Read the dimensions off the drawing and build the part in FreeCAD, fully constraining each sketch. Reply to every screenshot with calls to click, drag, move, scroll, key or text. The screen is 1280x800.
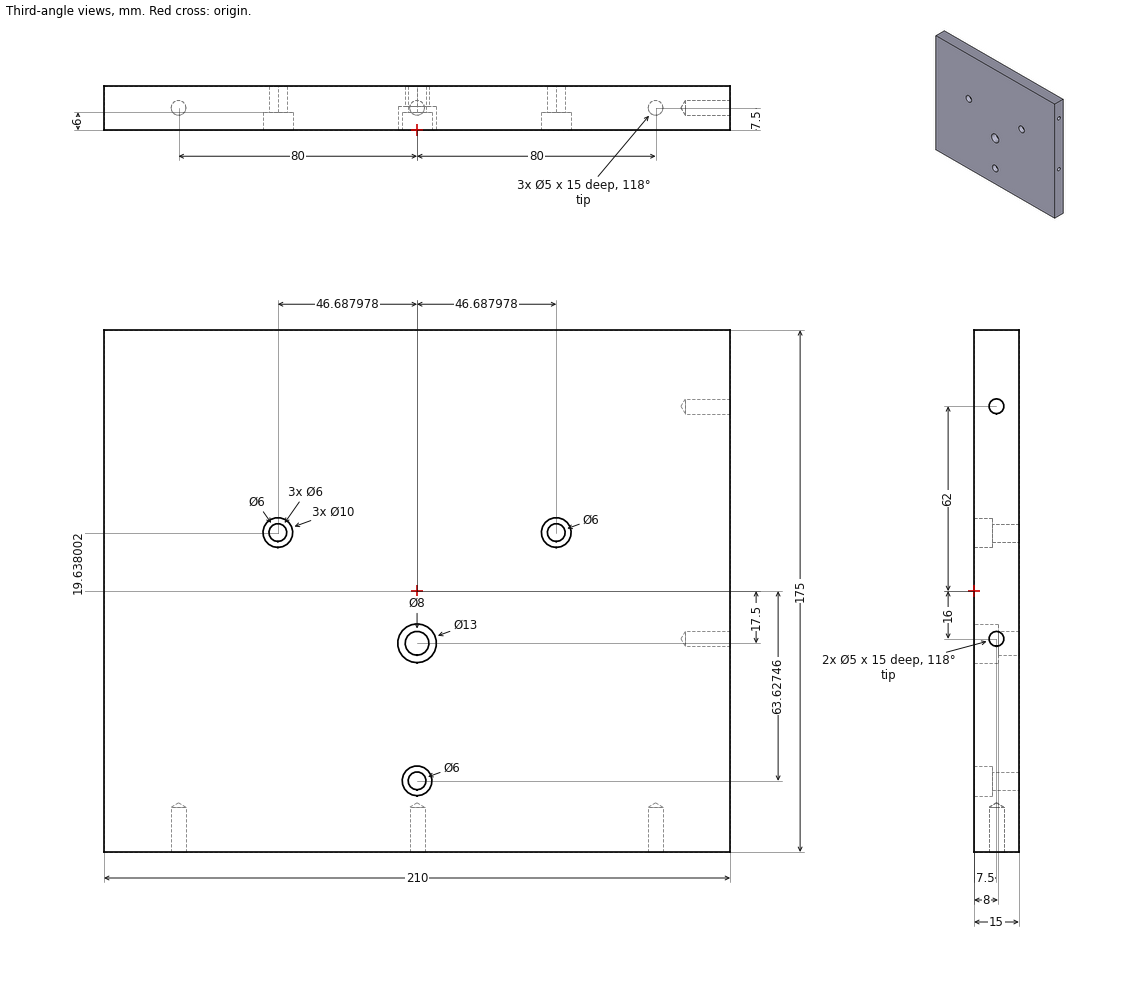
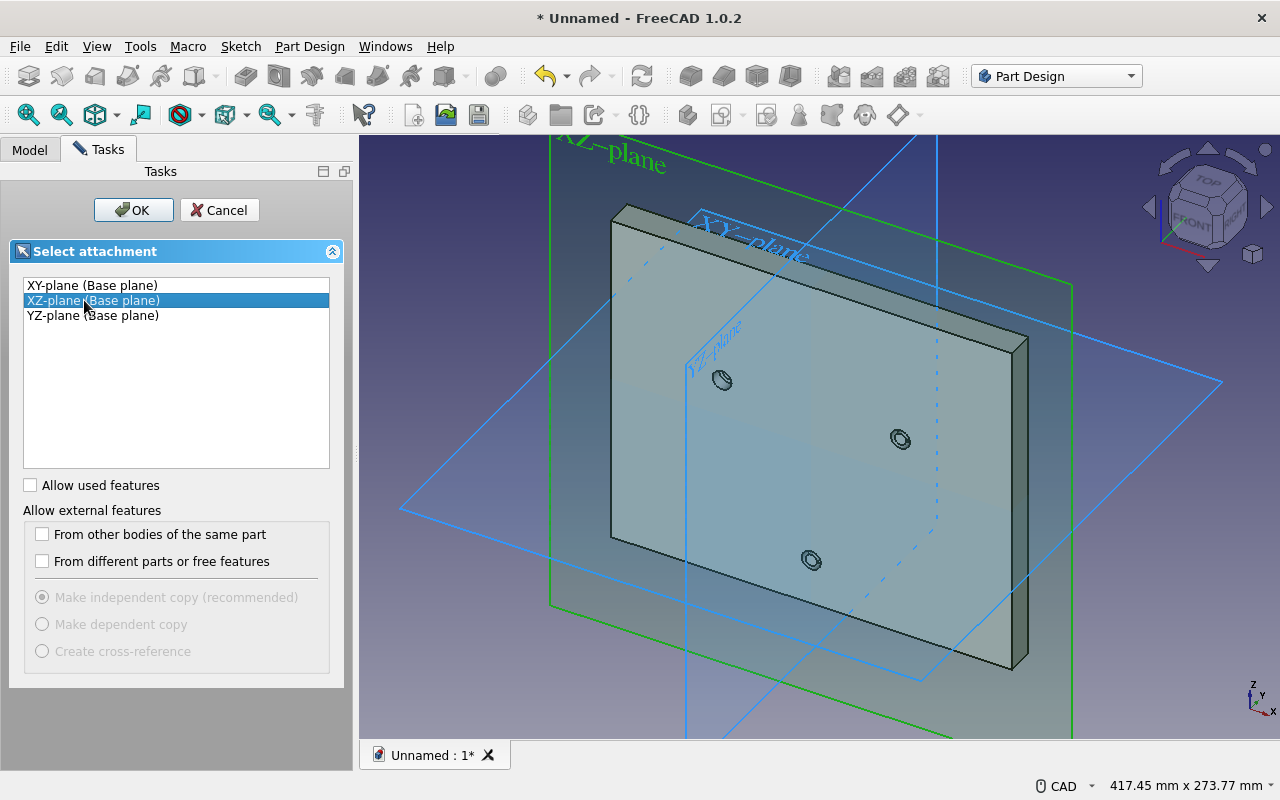
click(134, 210)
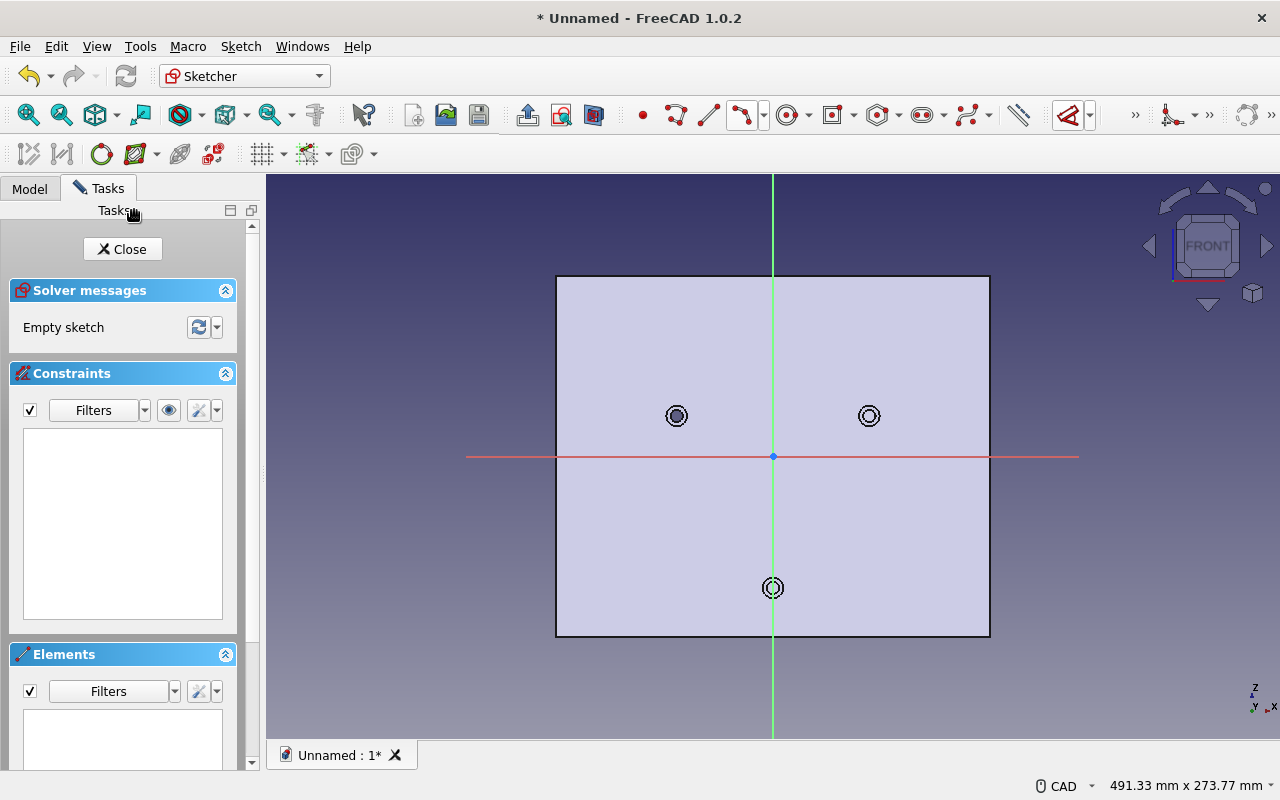
scroll(878, 414, up, 15)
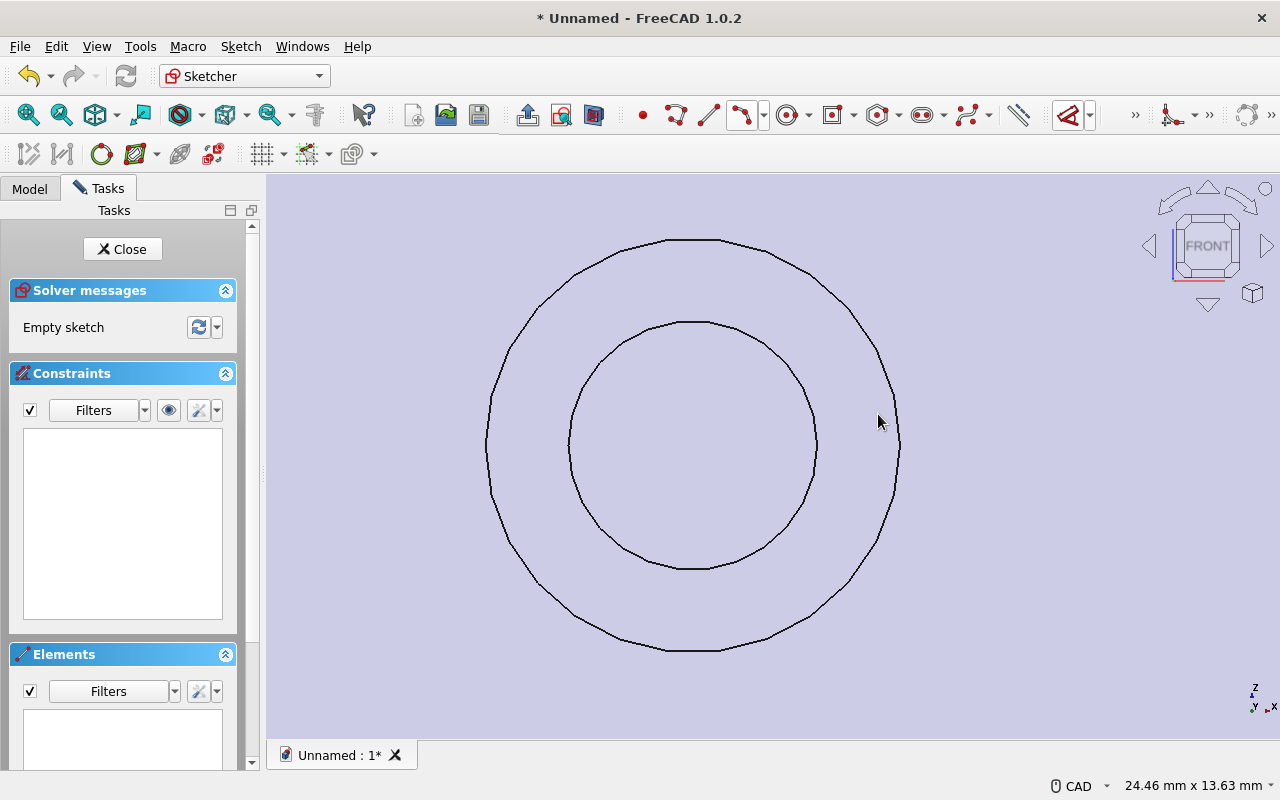
scroll(669, 423, up, 2)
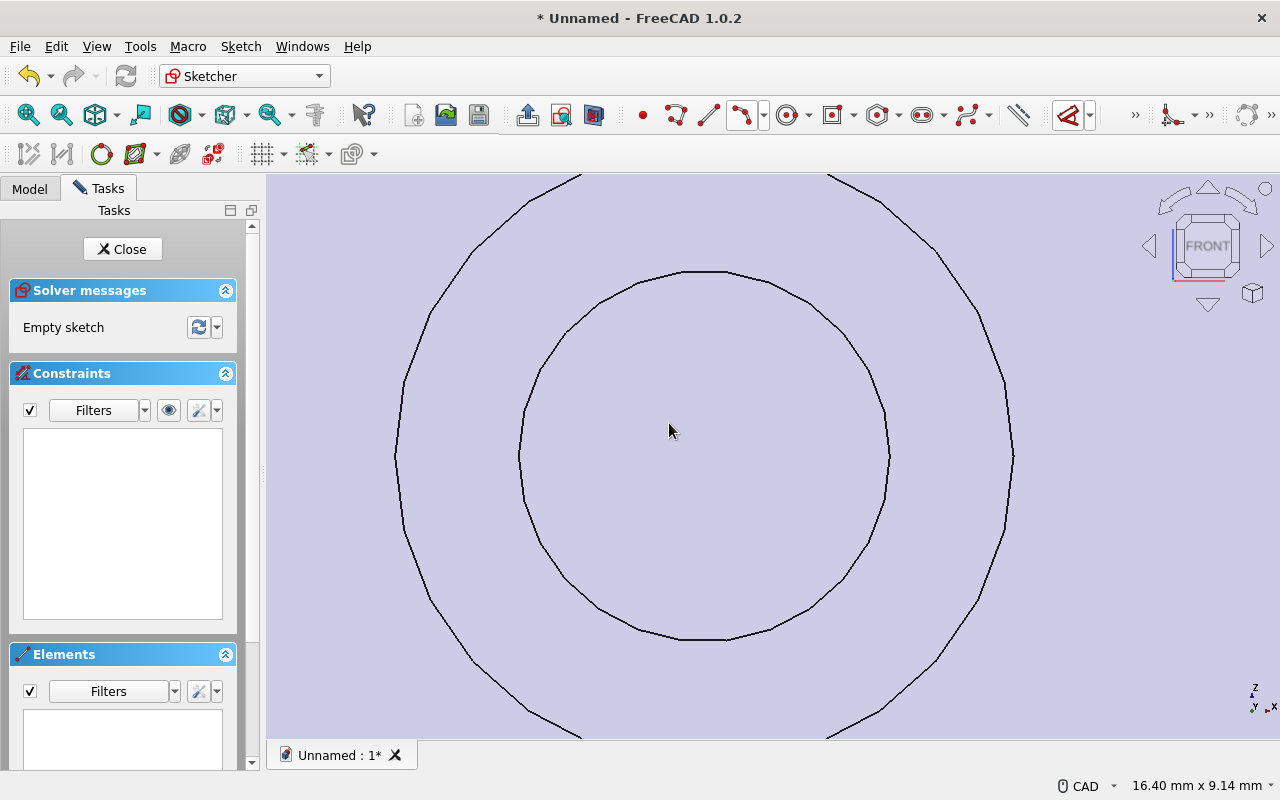
click(786, 116)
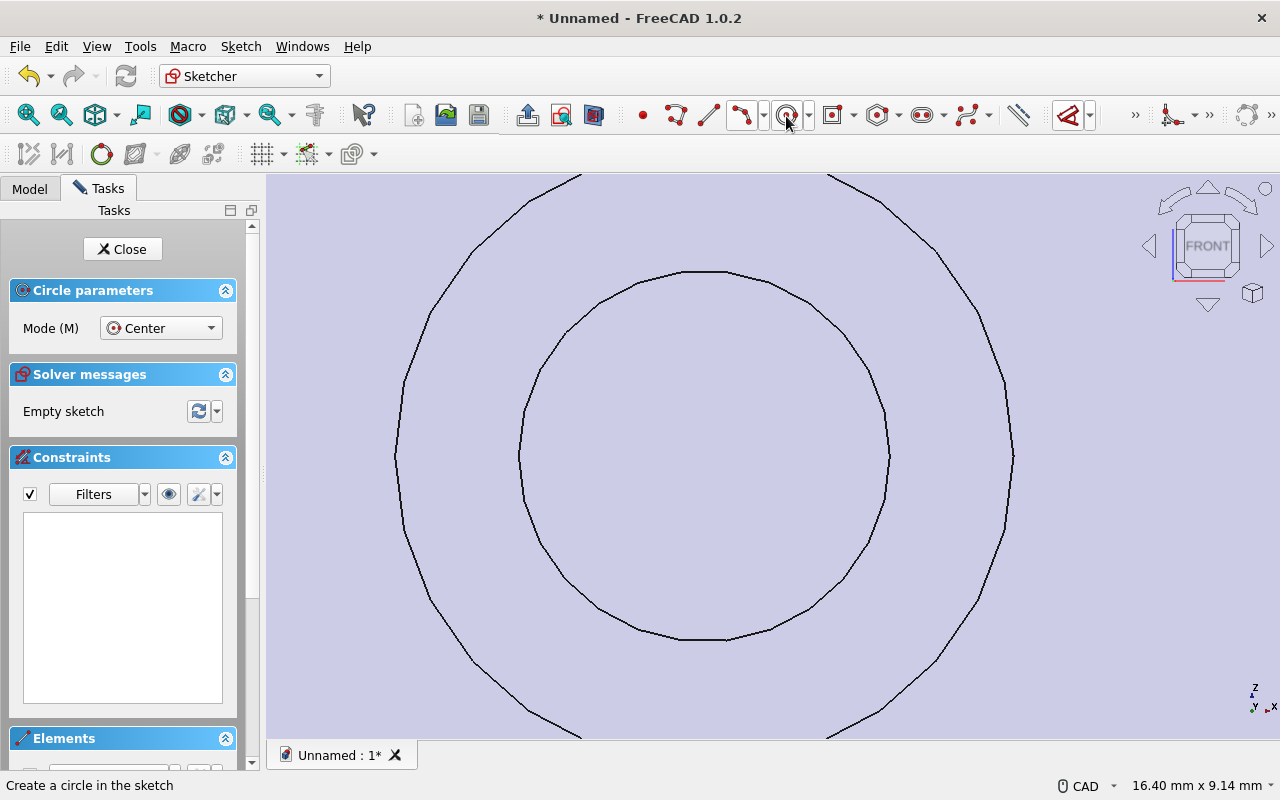
click(704, 456)
click(835, 325)
key(Escape)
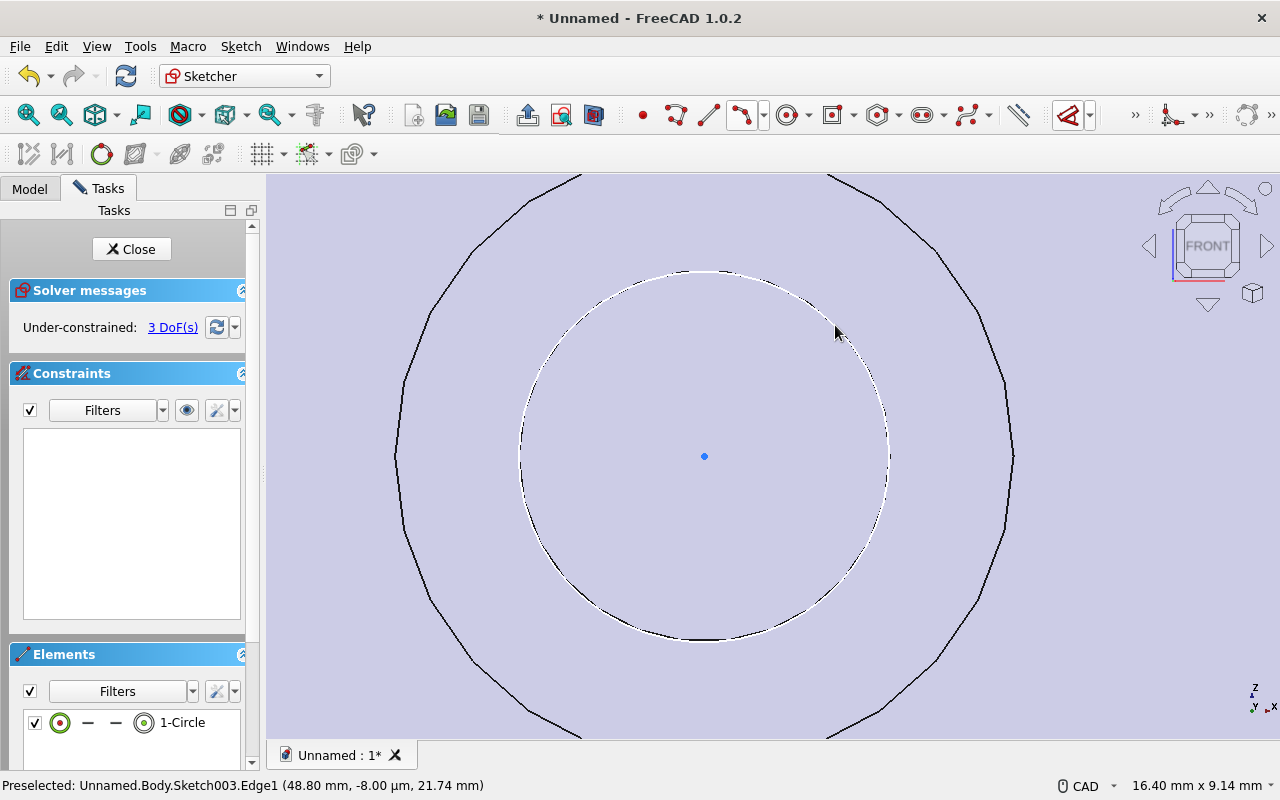
click(835, 326)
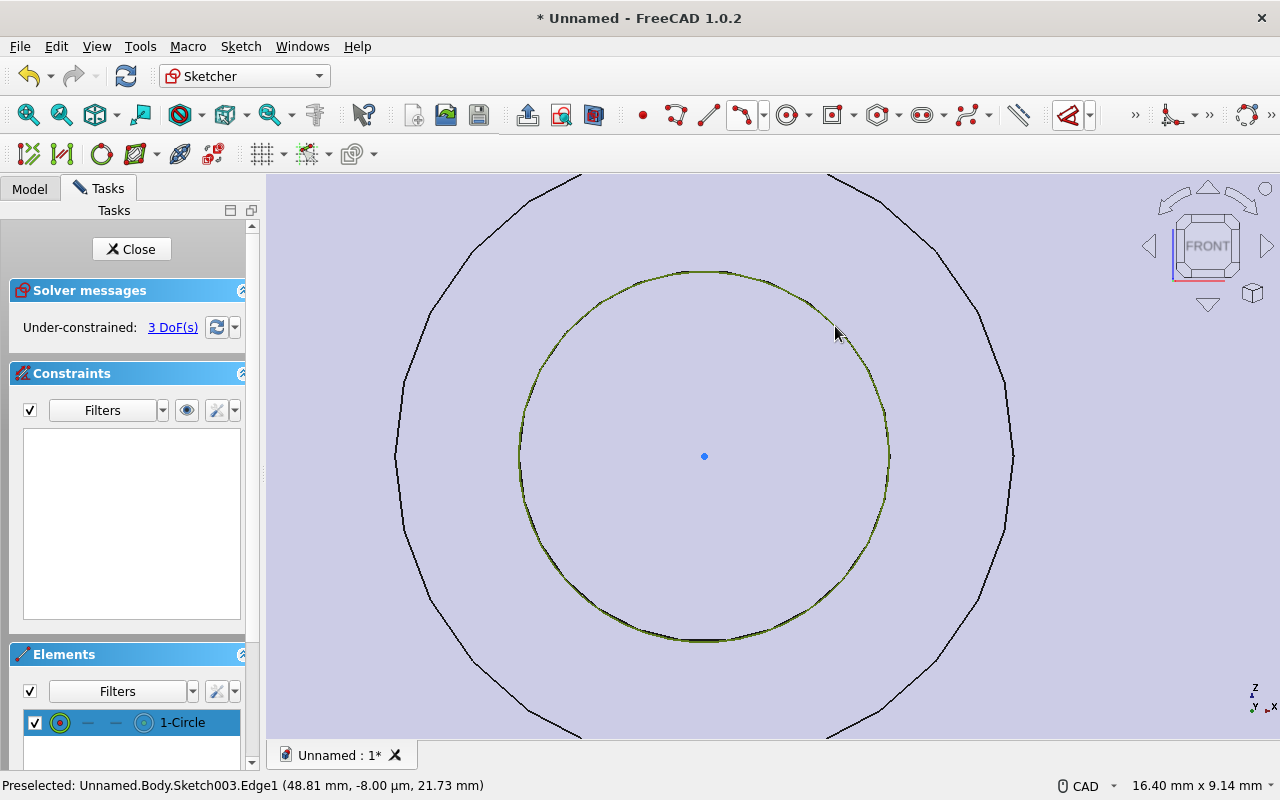
key(k)
key(o)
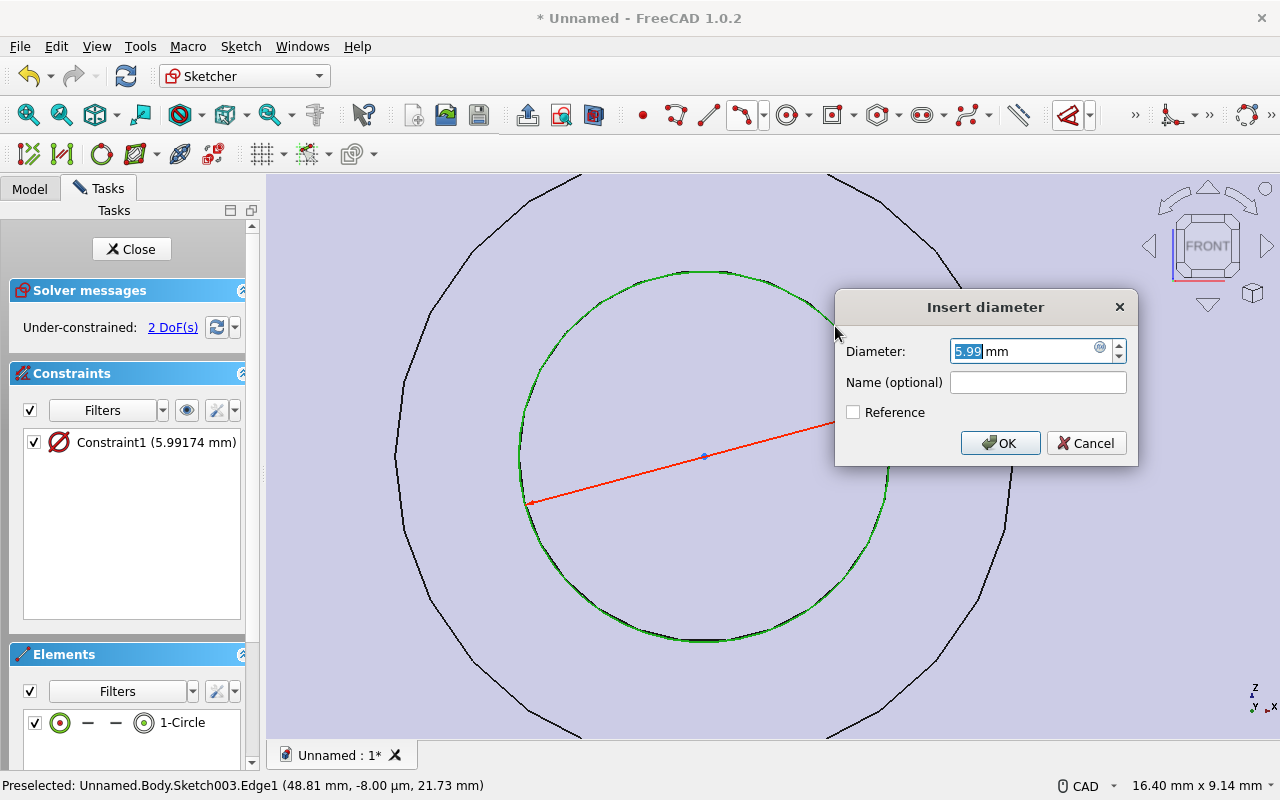
text(6)
key(Return)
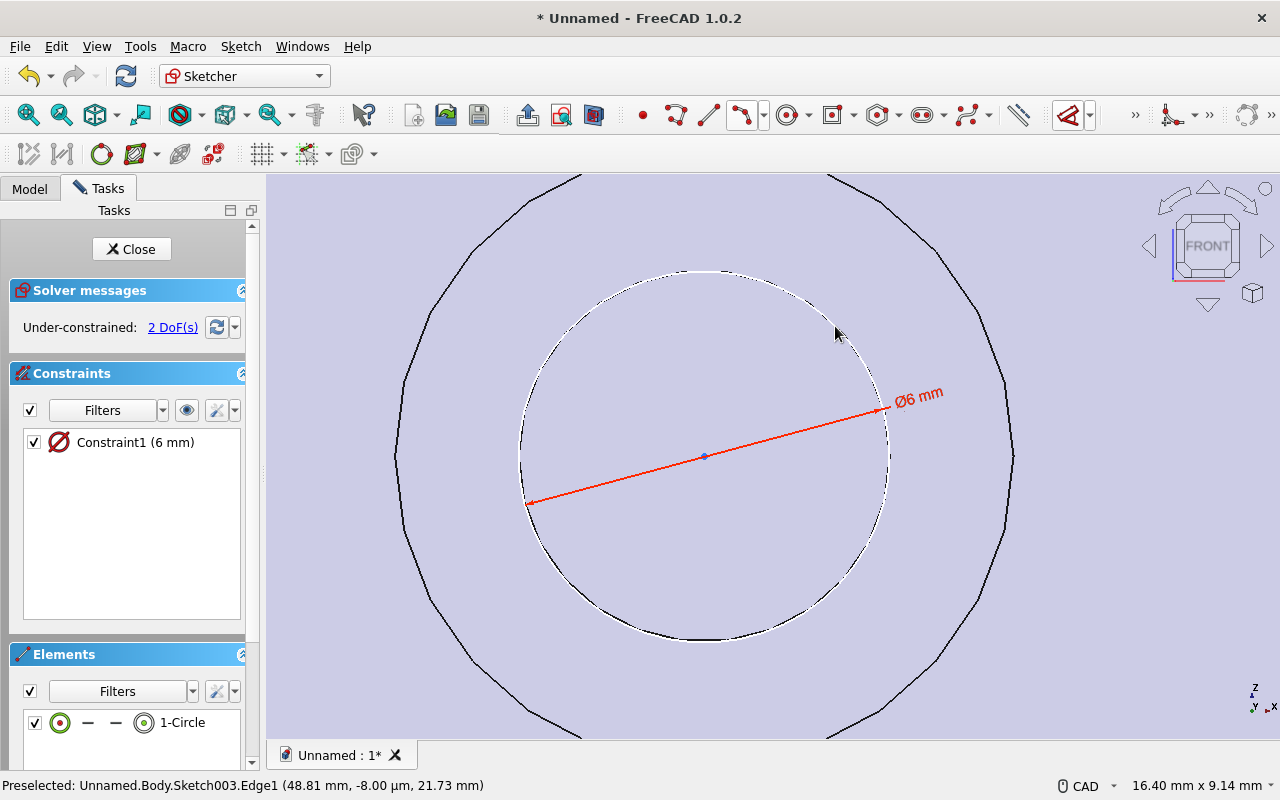
click(704, 457)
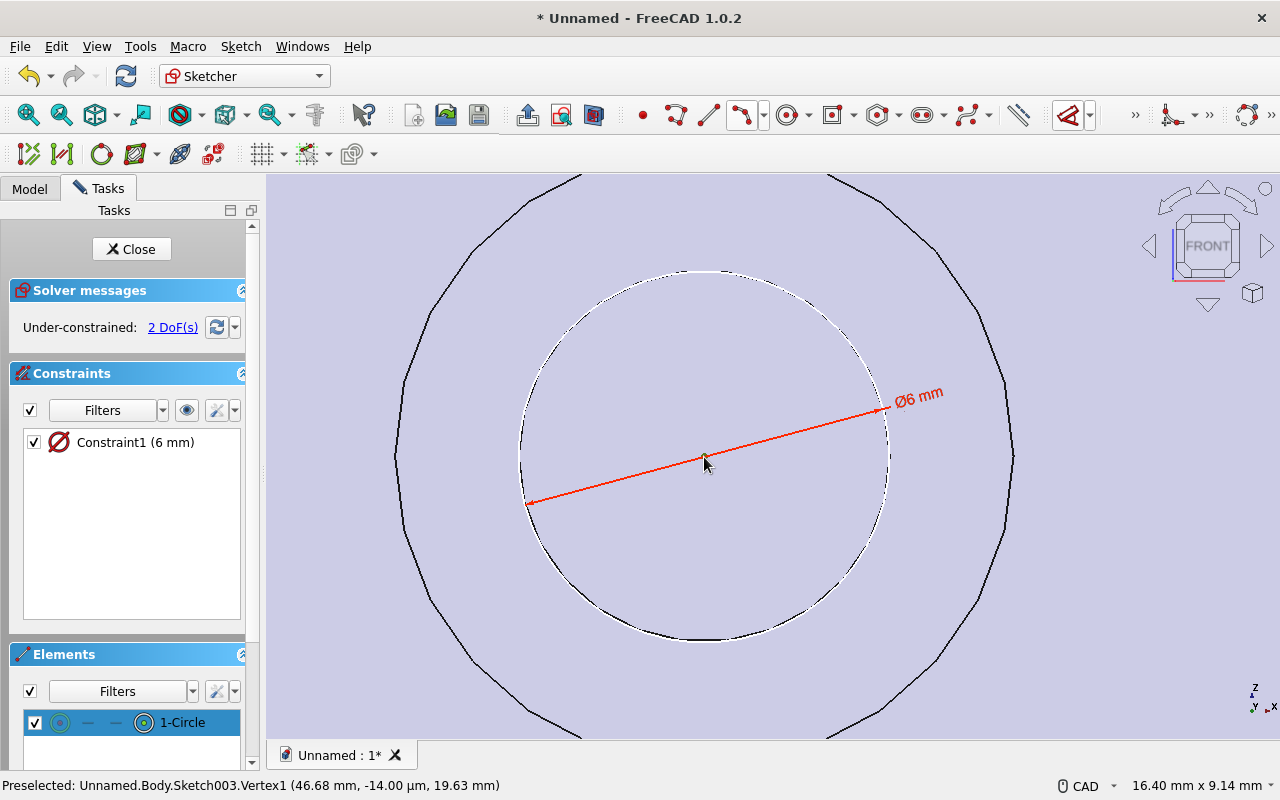
key(l)